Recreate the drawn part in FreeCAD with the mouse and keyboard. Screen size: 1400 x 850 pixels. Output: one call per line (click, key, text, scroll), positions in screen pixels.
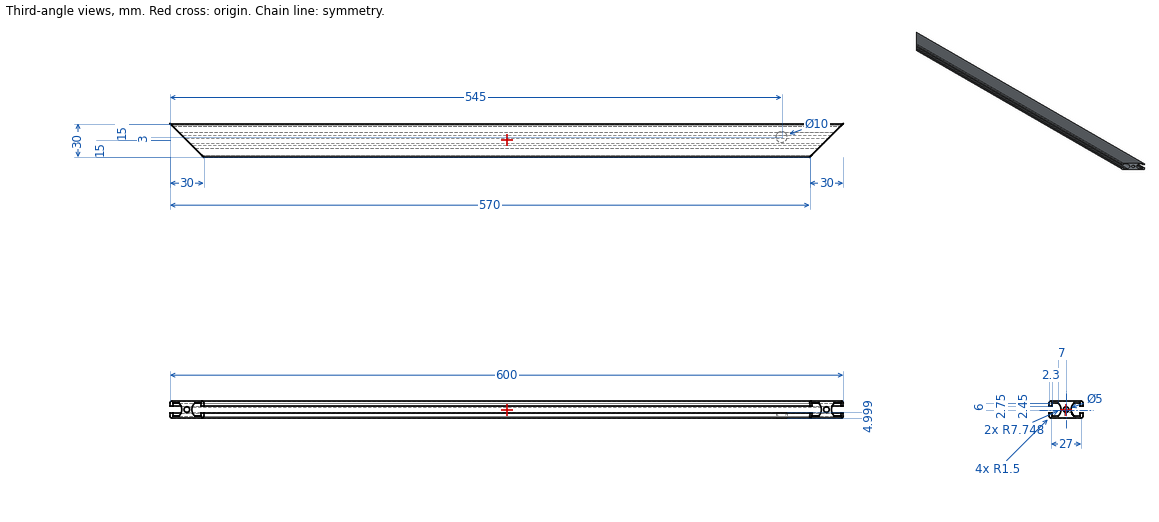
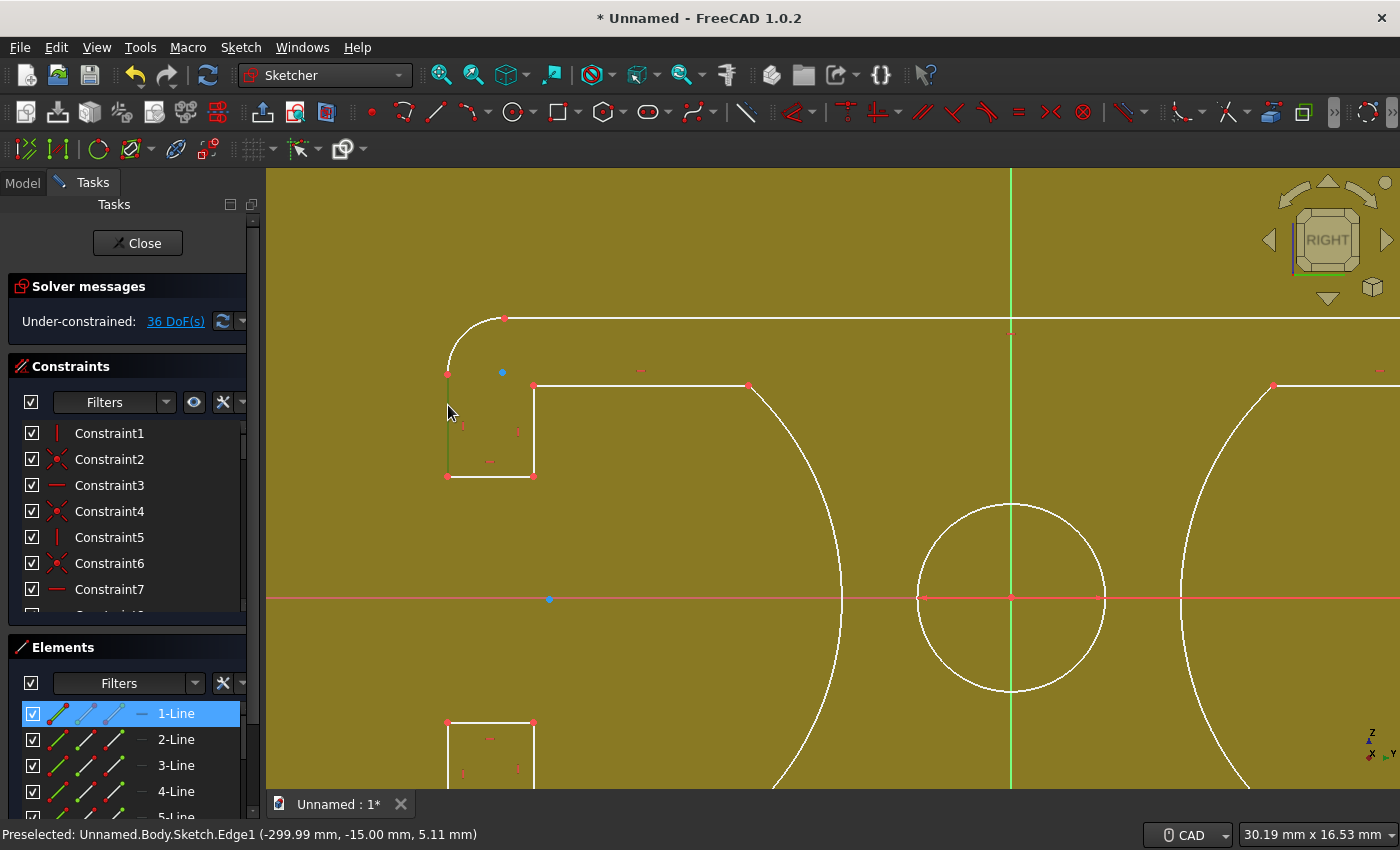
click(478, 324)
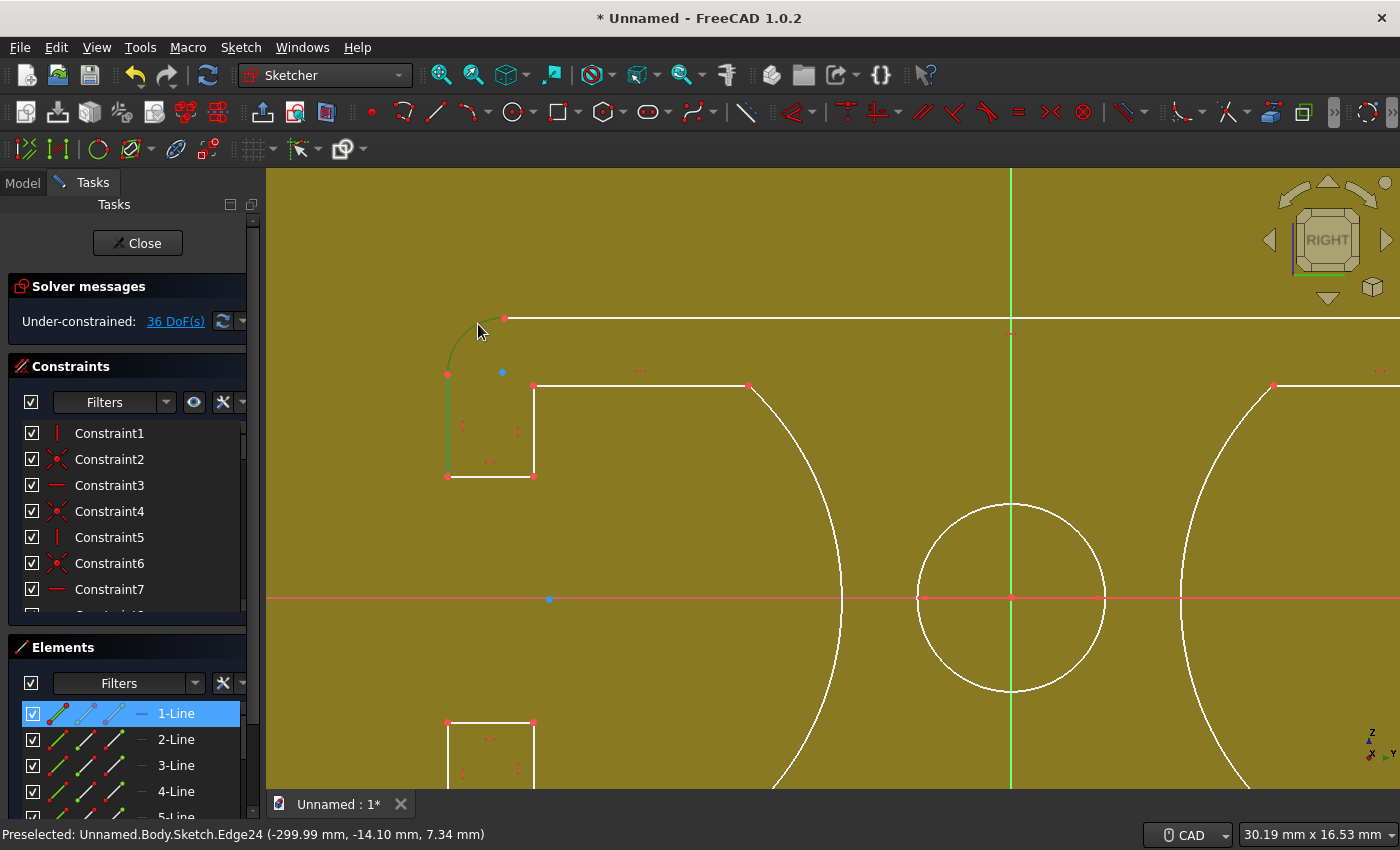
key(t)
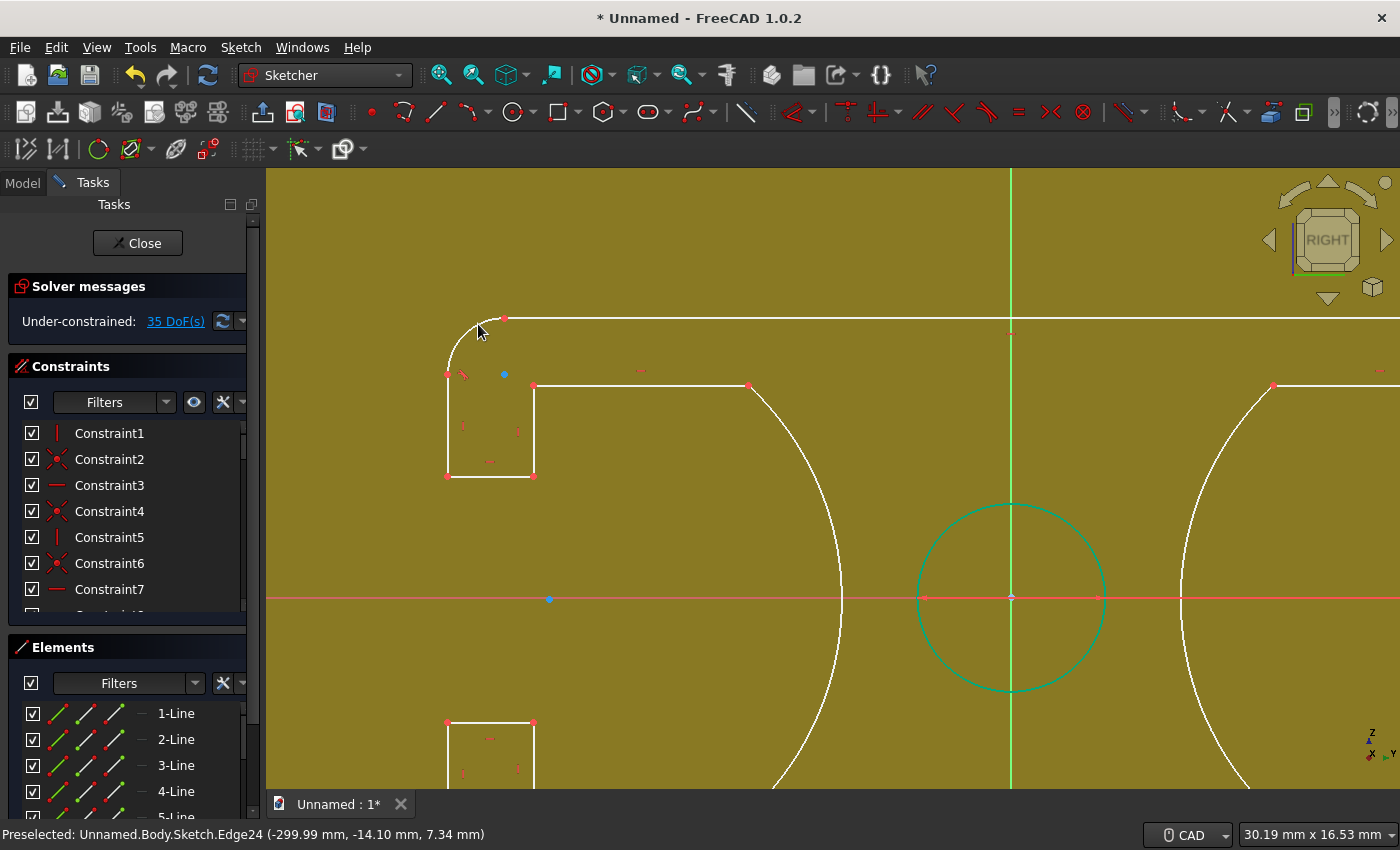
click(448, 753)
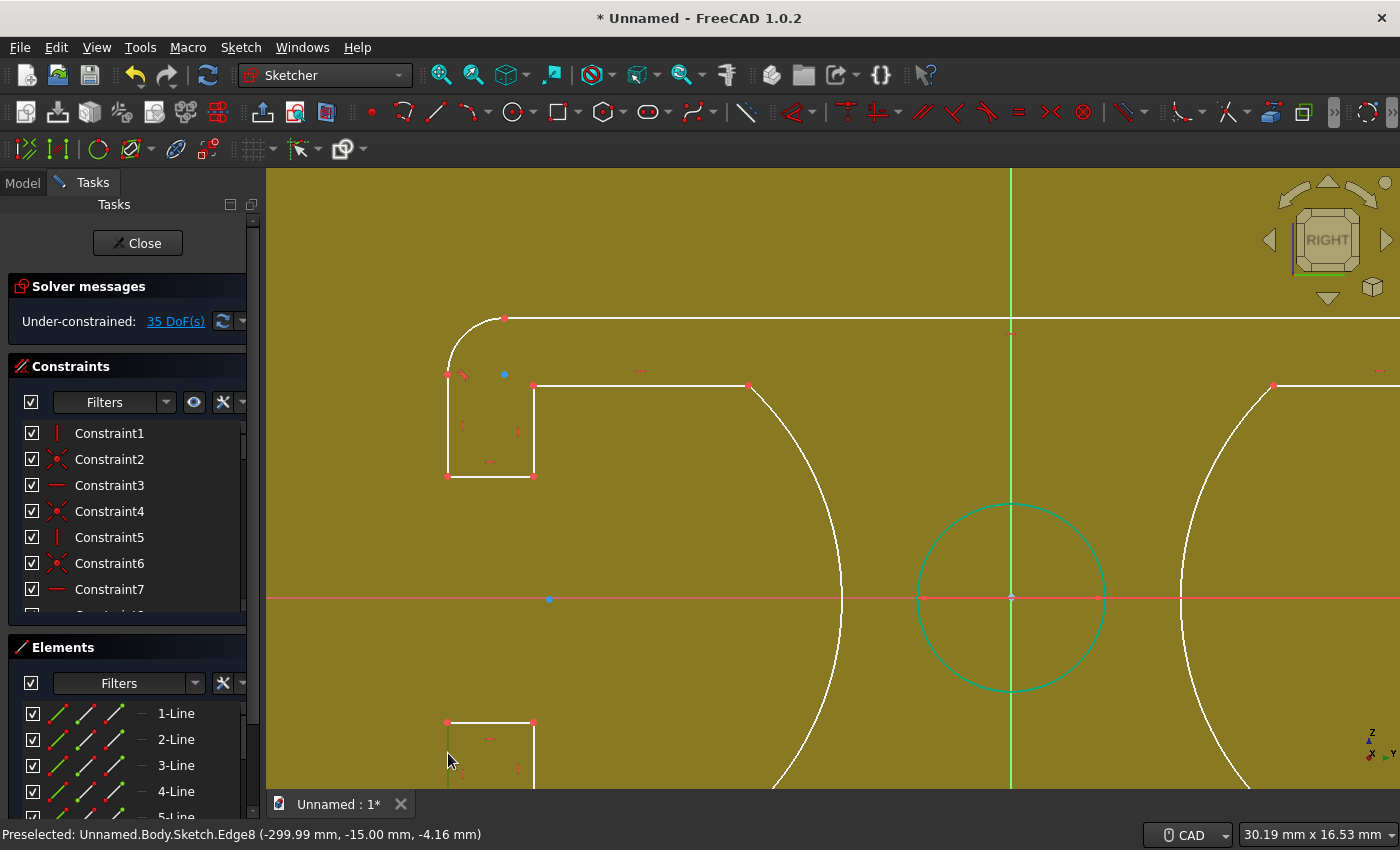
scroll(464, 333, down, 3)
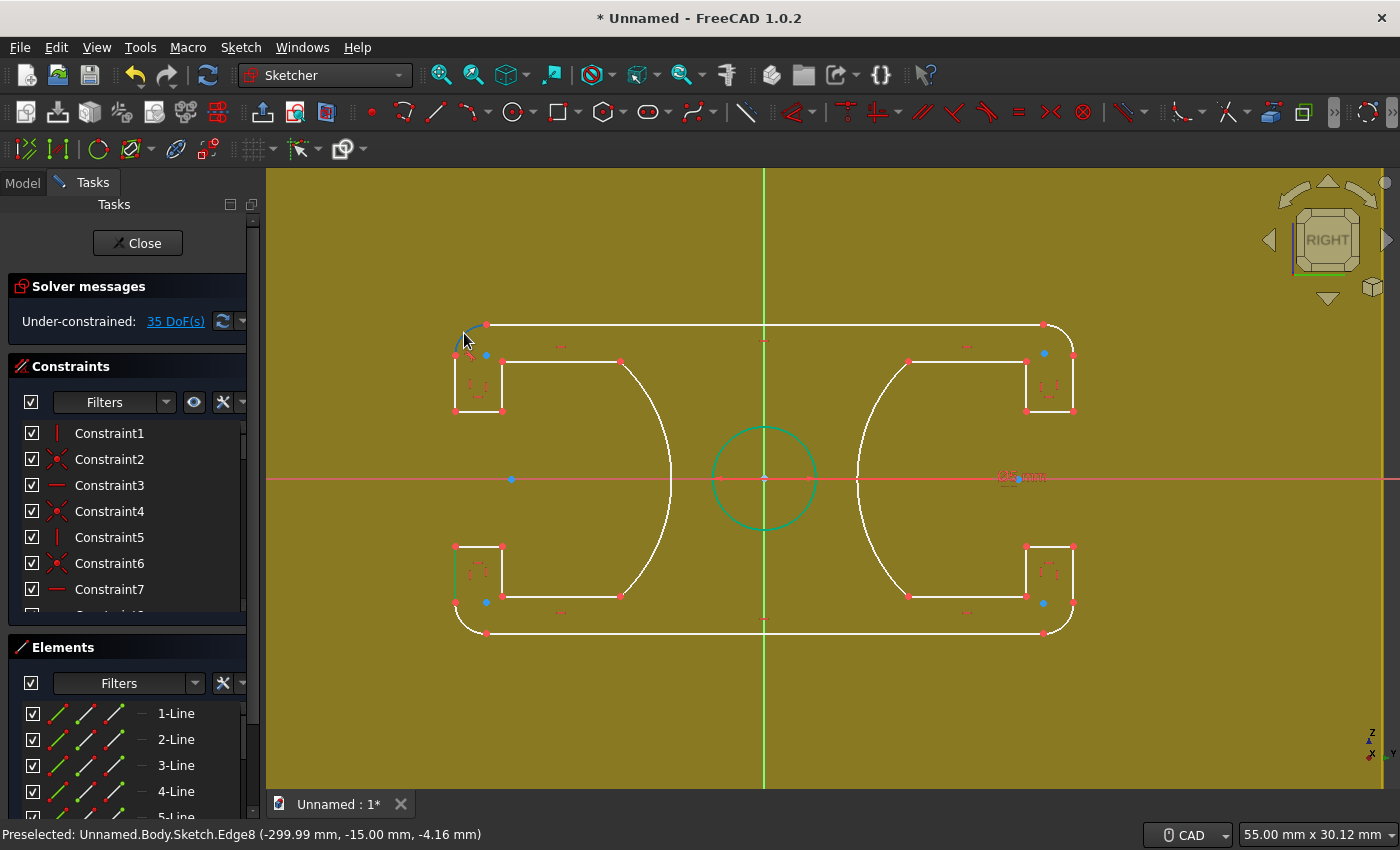
click(459, 617)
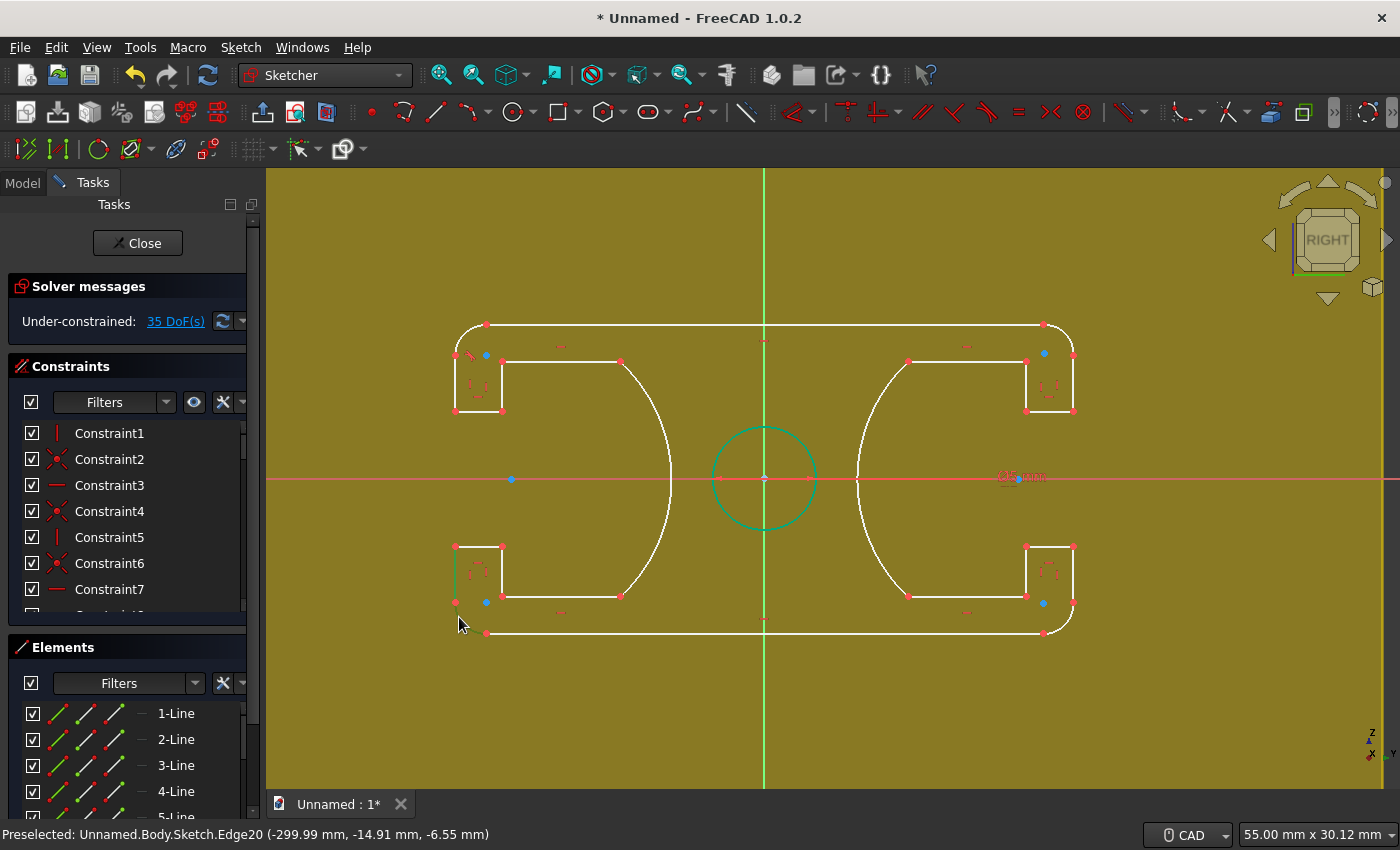
key(t)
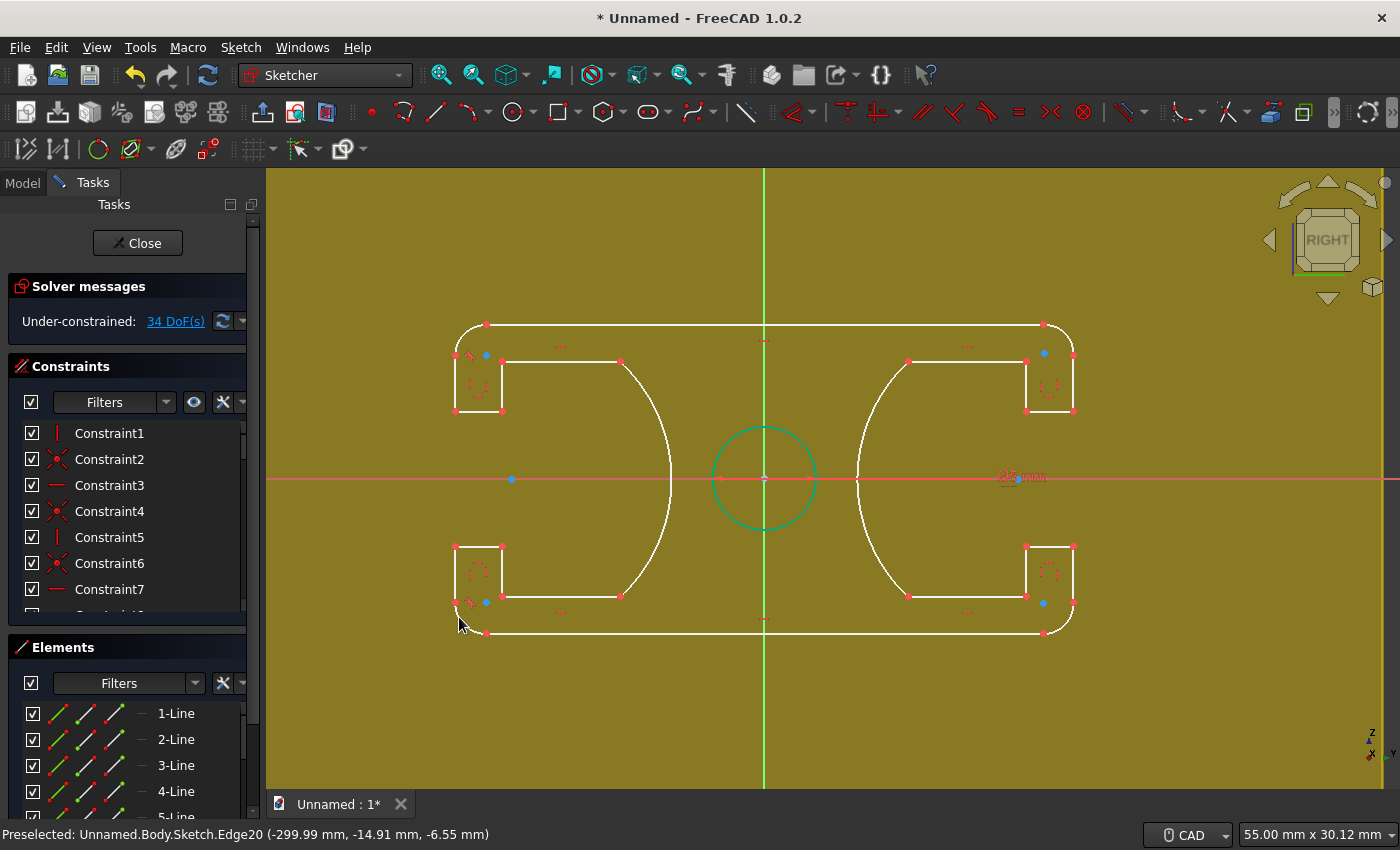
click(653, 634)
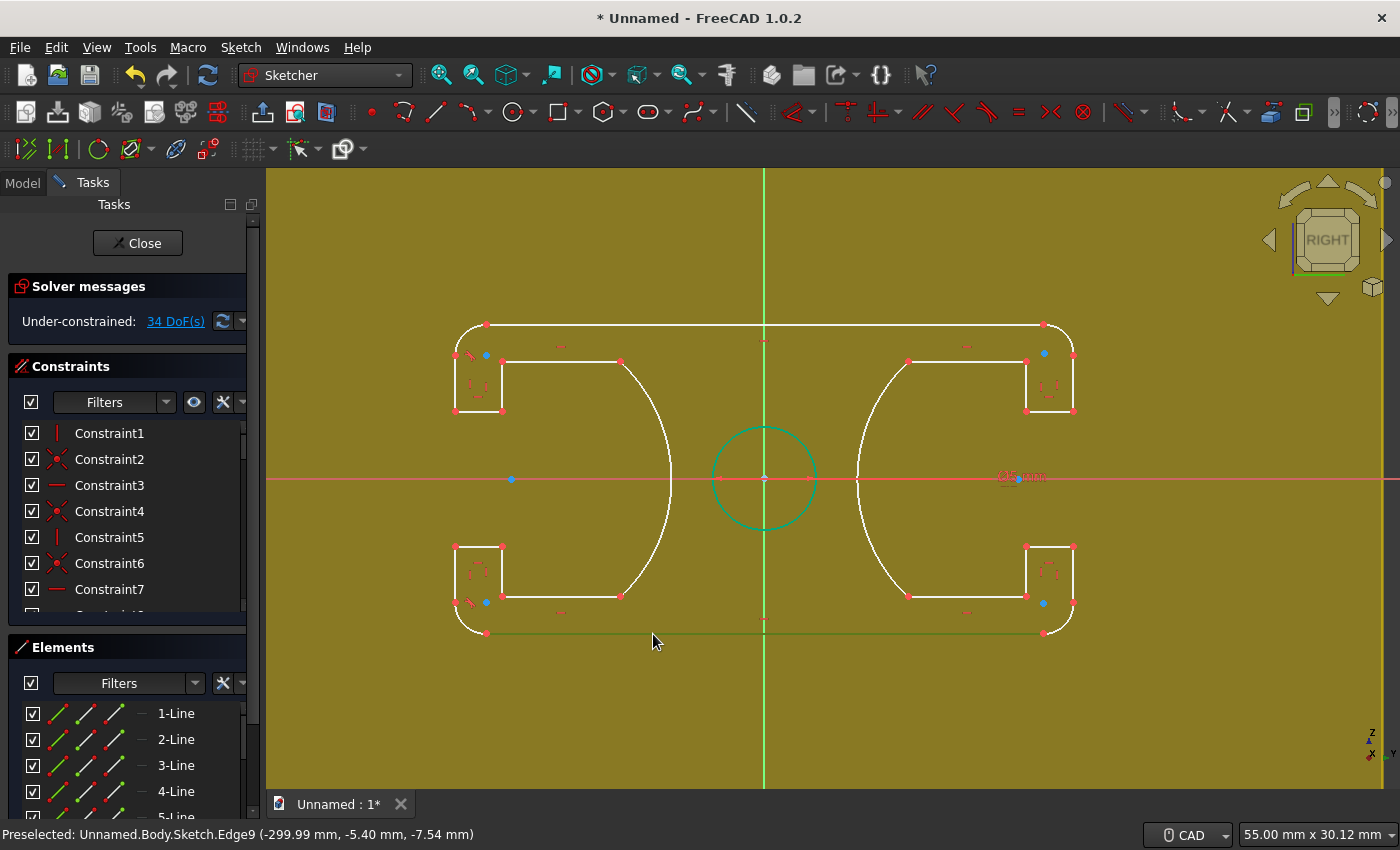
click(459, 617)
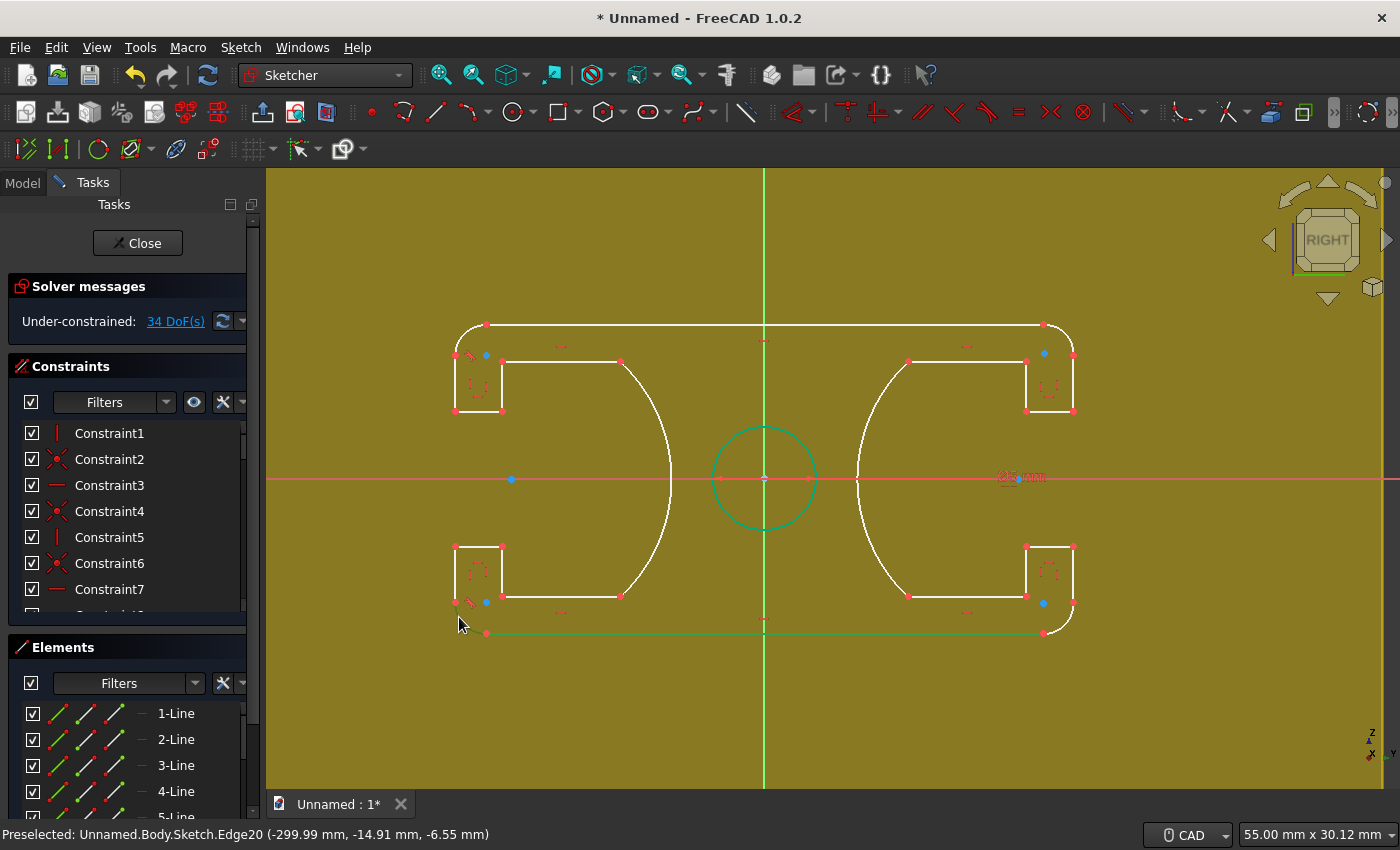
key(t)